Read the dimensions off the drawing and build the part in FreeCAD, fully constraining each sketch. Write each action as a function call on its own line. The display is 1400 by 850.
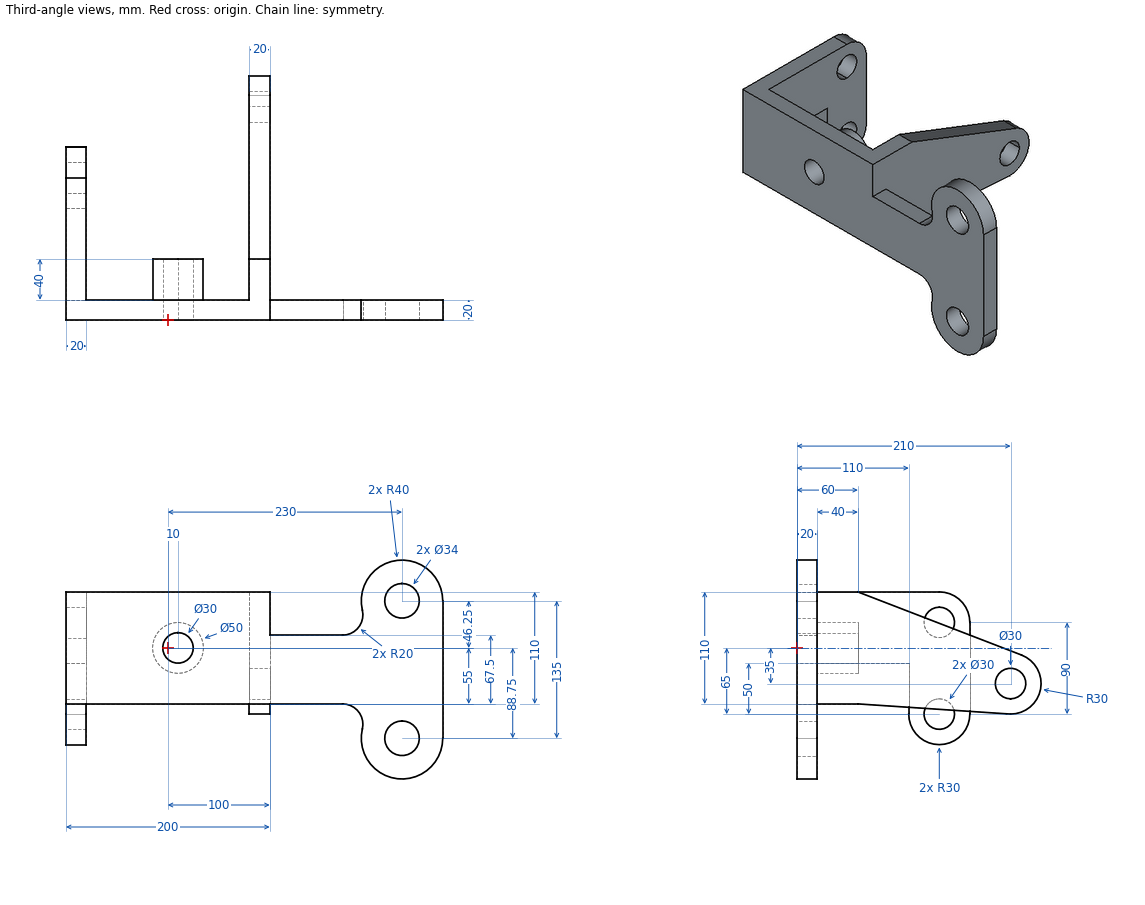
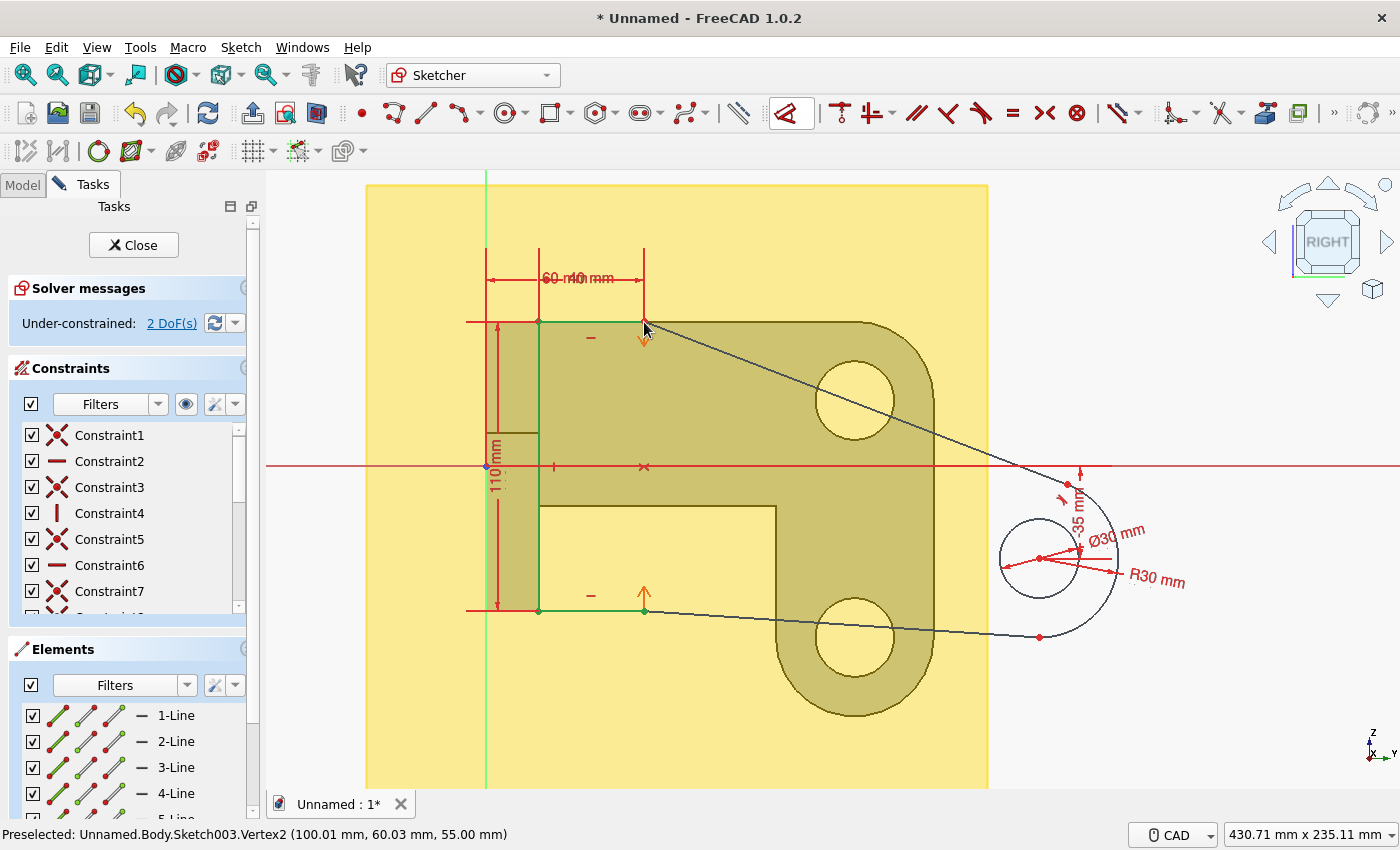
click(1039, 559)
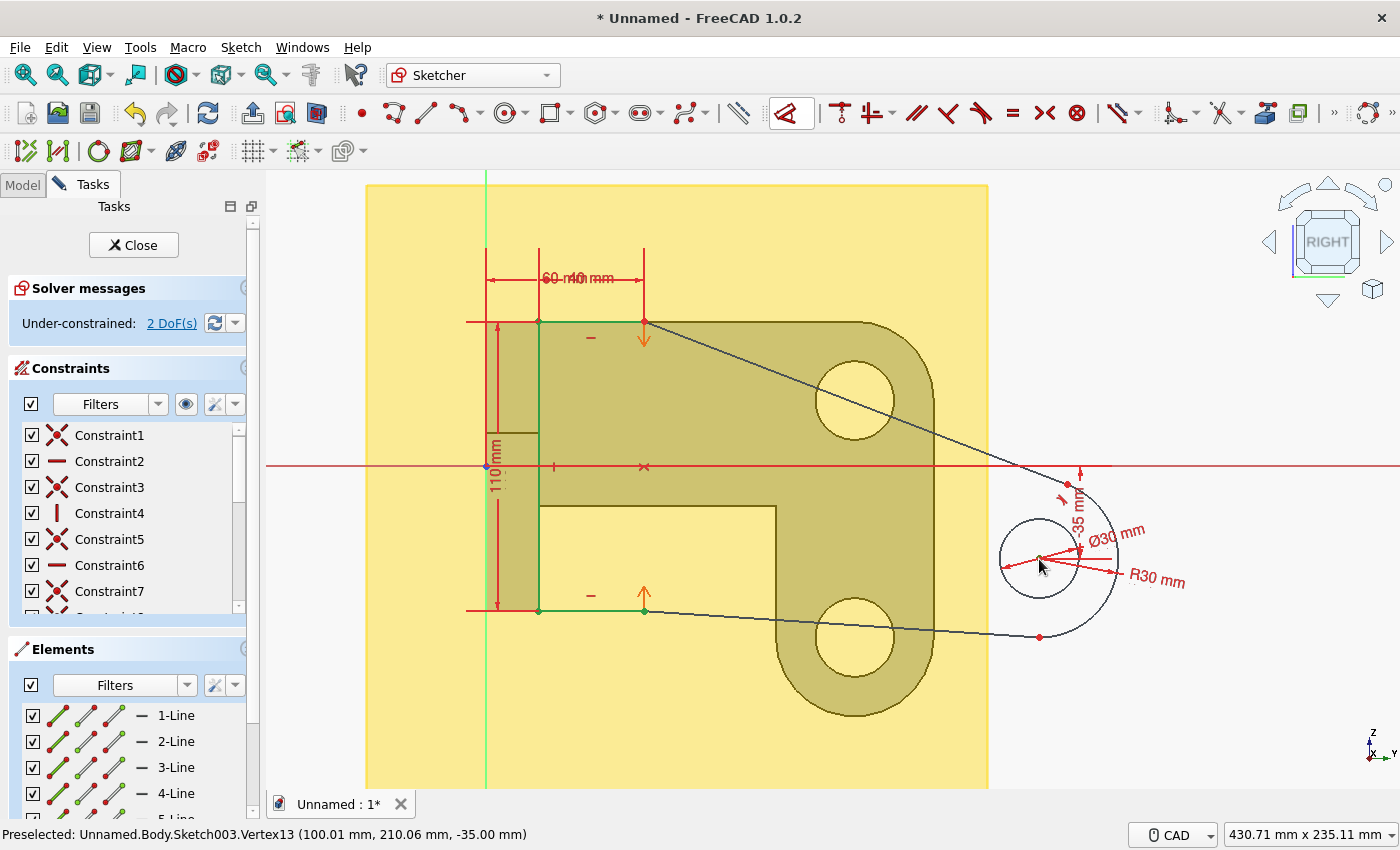
click(808, 114)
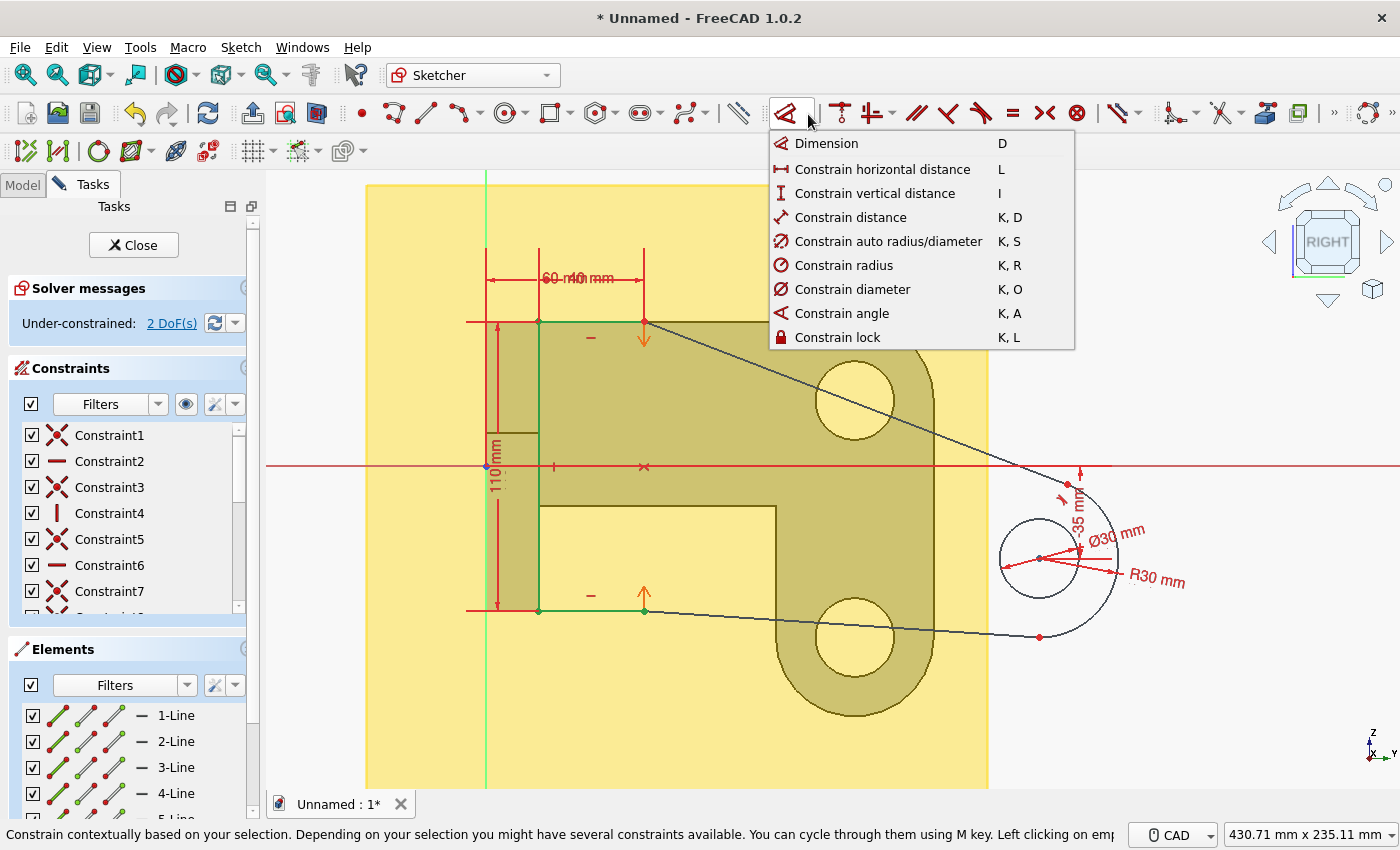
click(922, 169)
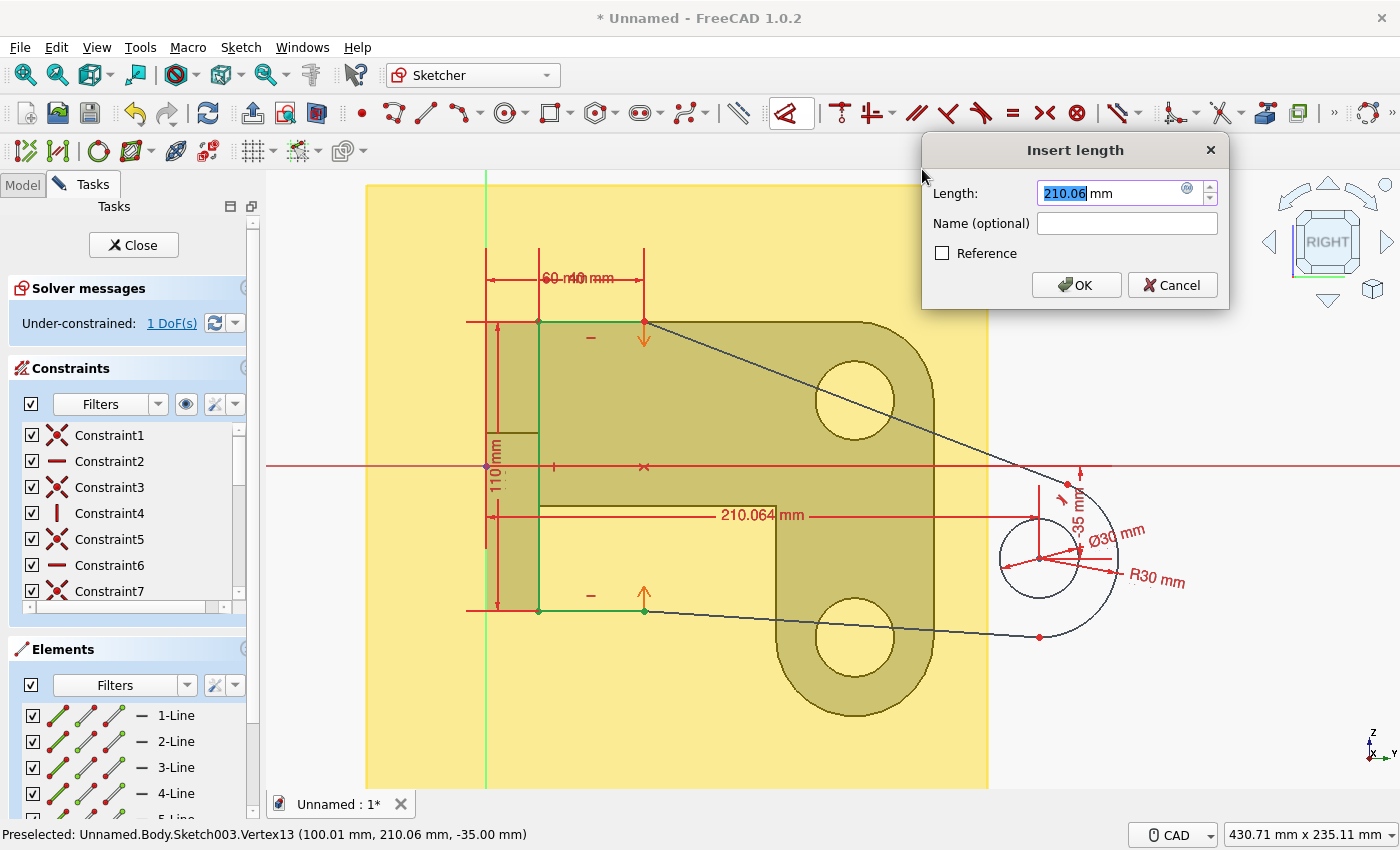
text(210)
key(Return)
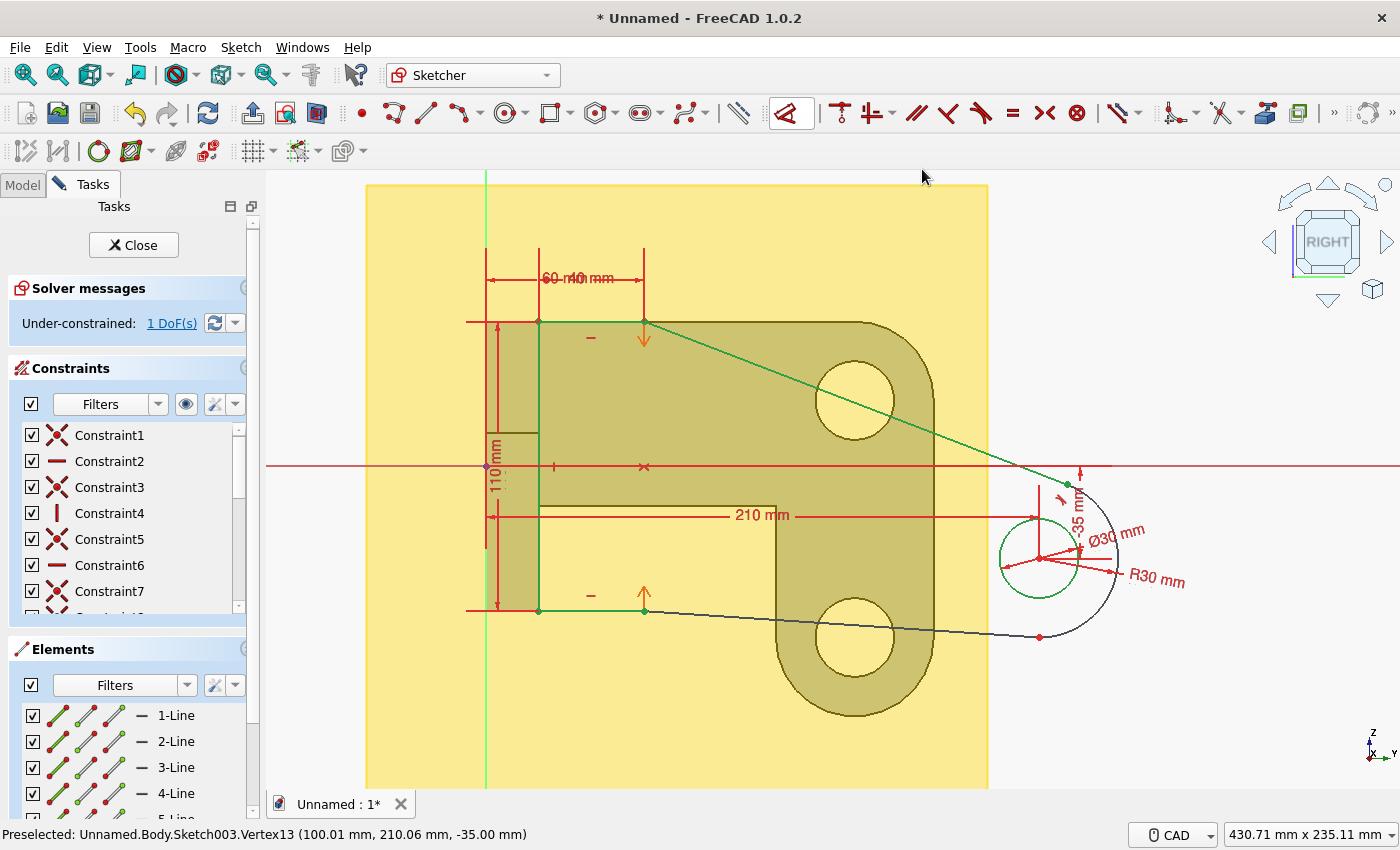
click(1039, 638)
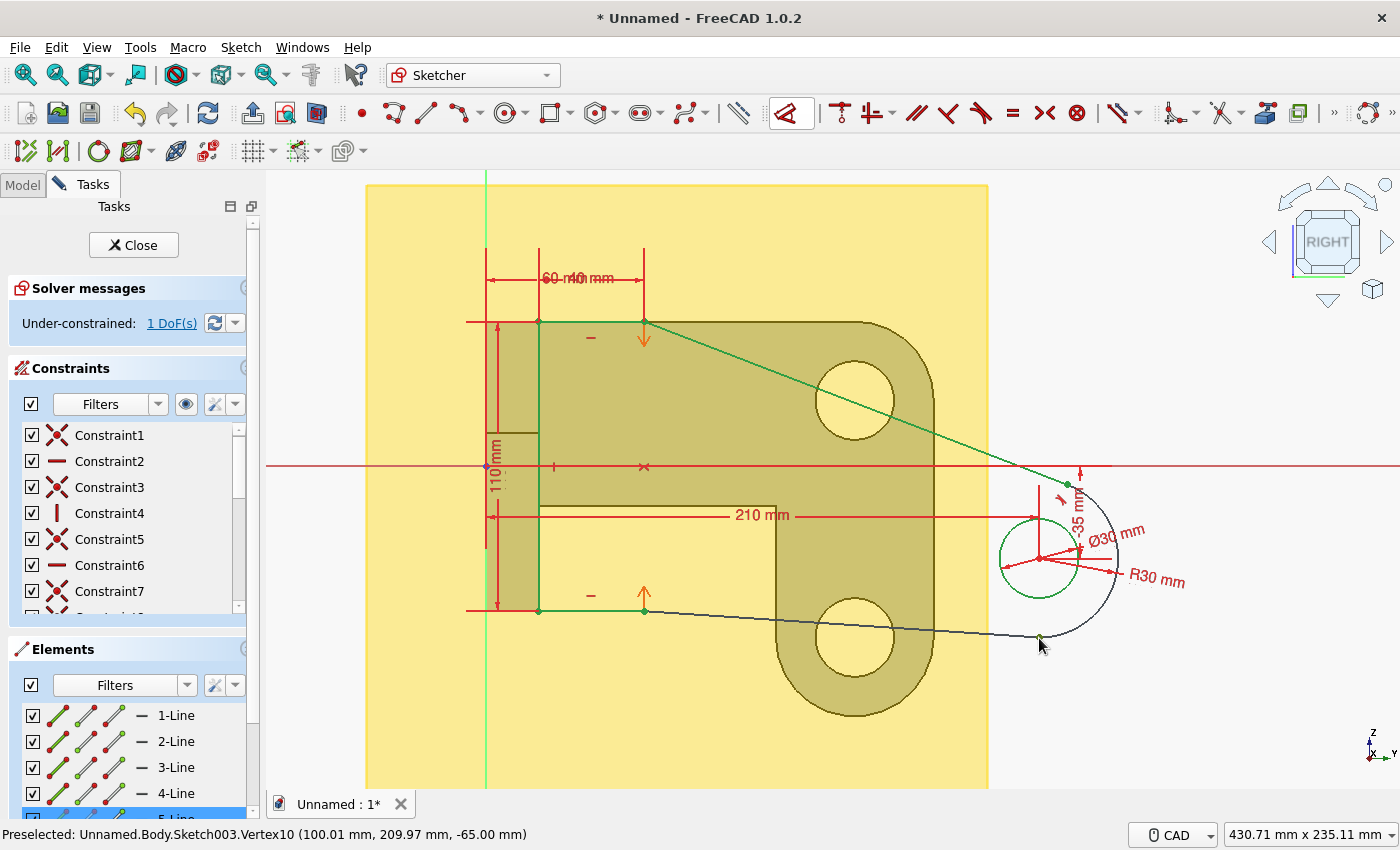
key(l)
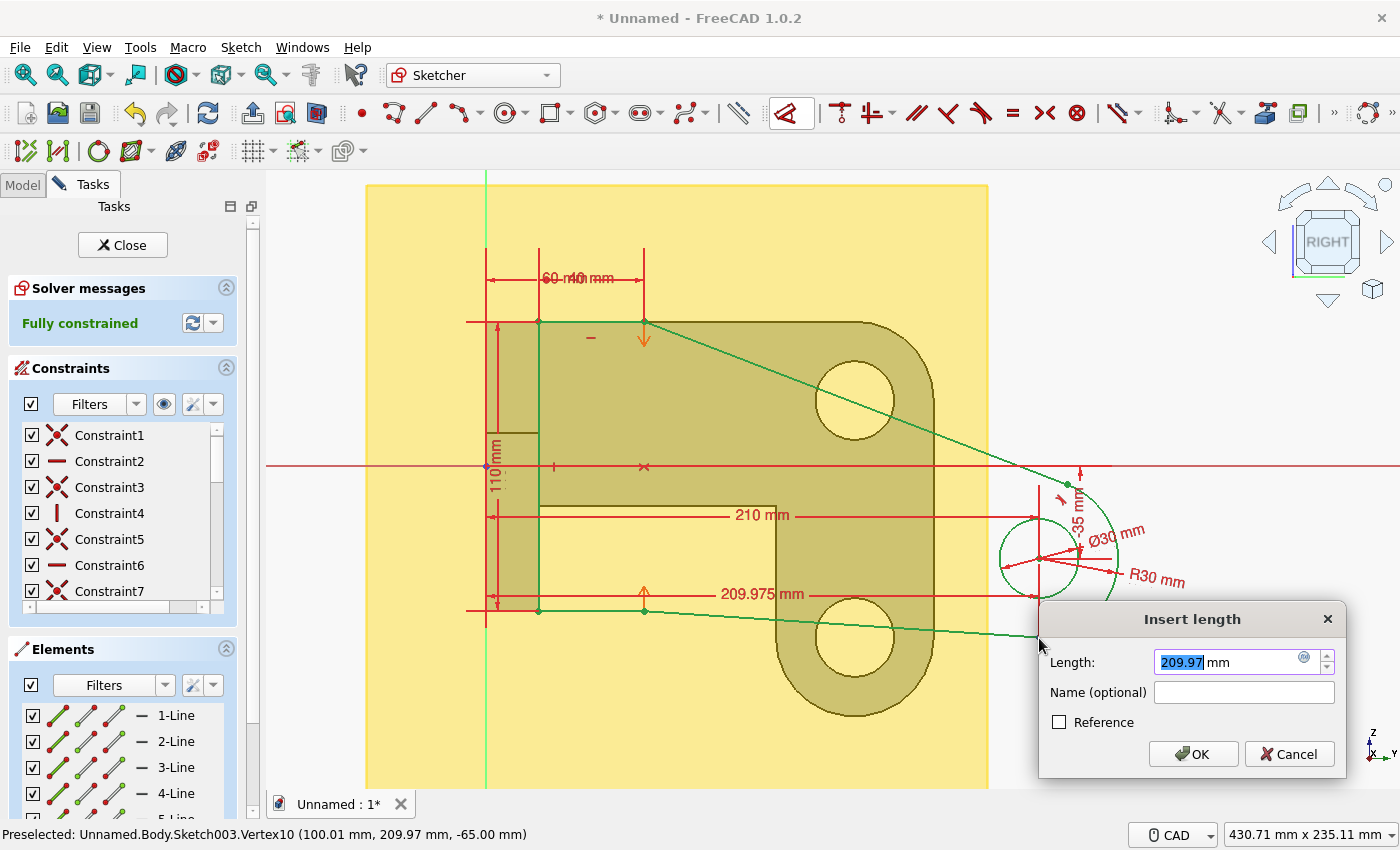
text(210)
key(Return)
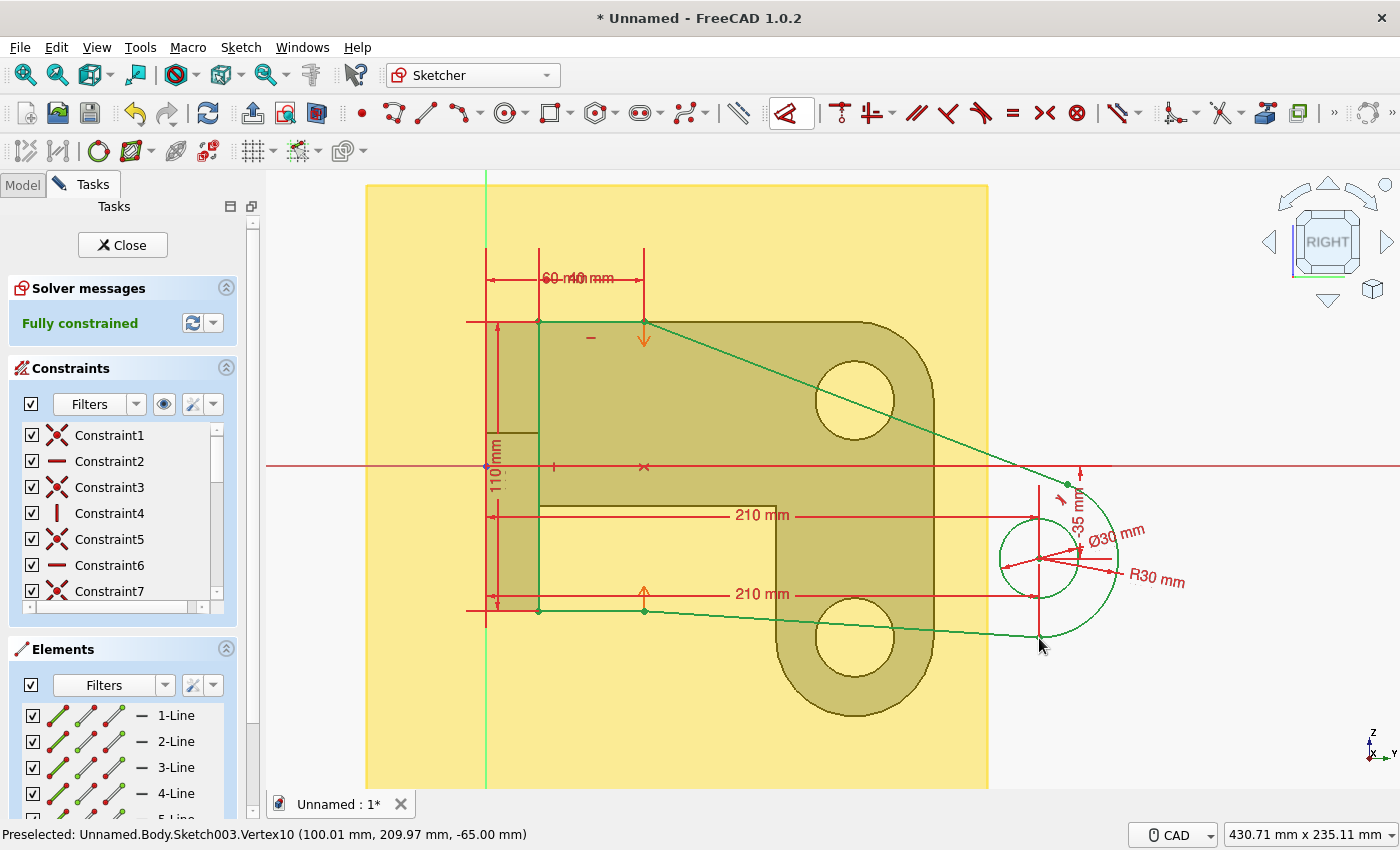
click(123, 245)